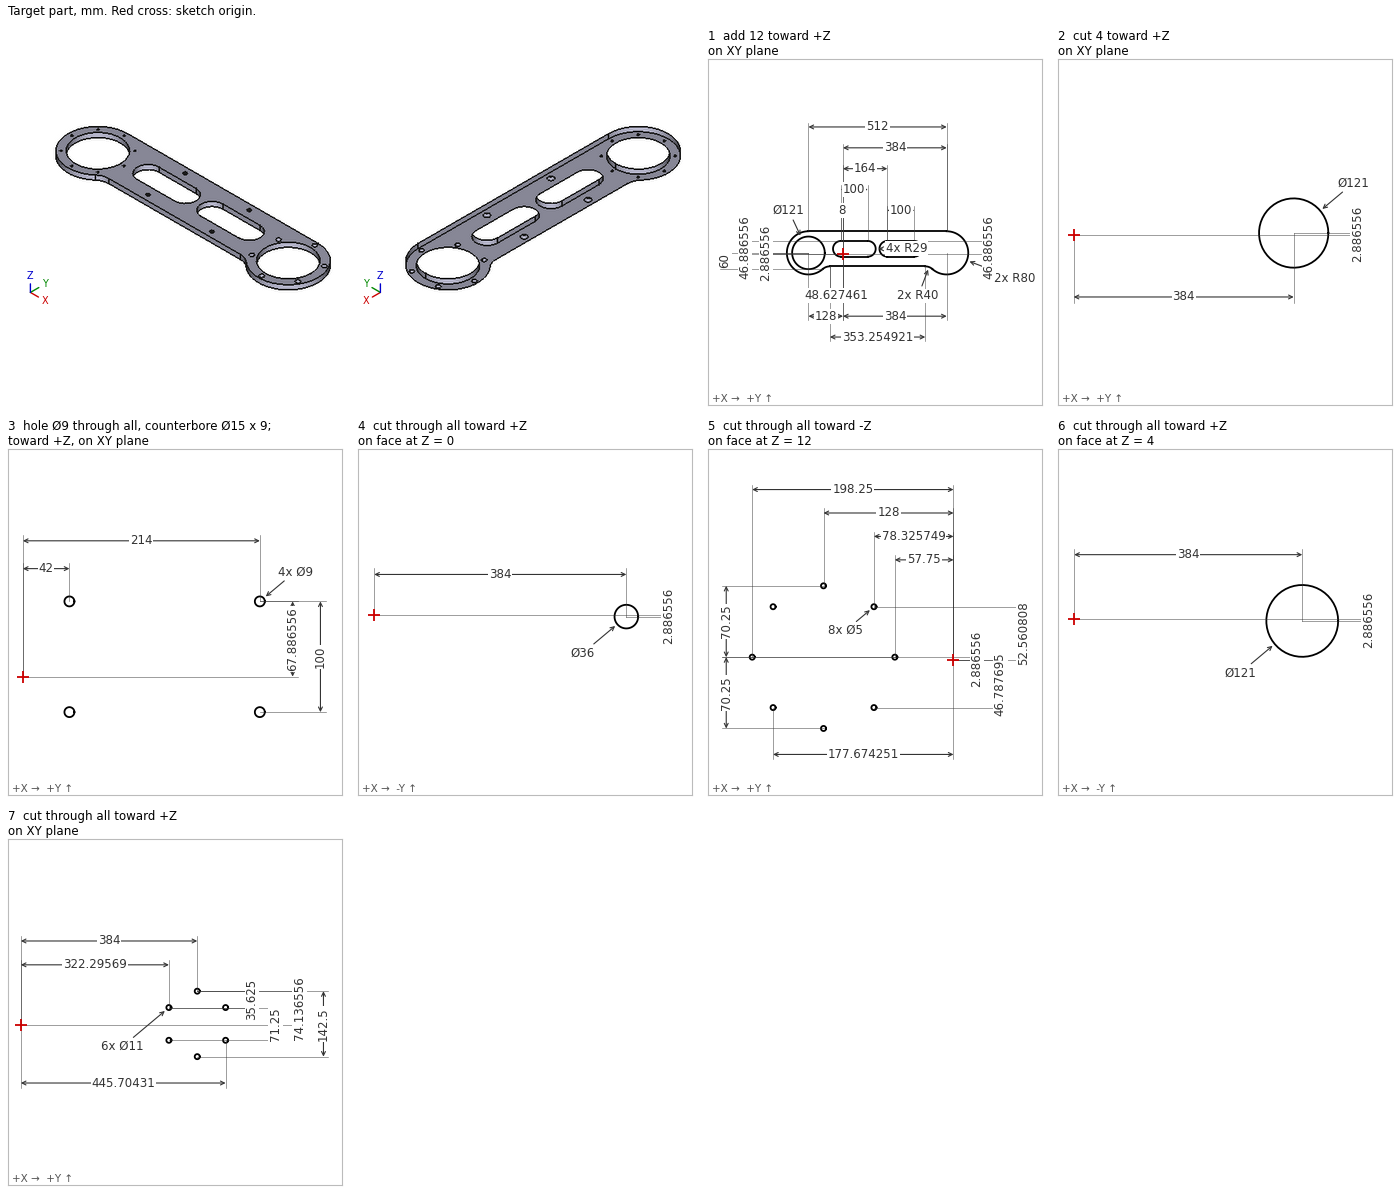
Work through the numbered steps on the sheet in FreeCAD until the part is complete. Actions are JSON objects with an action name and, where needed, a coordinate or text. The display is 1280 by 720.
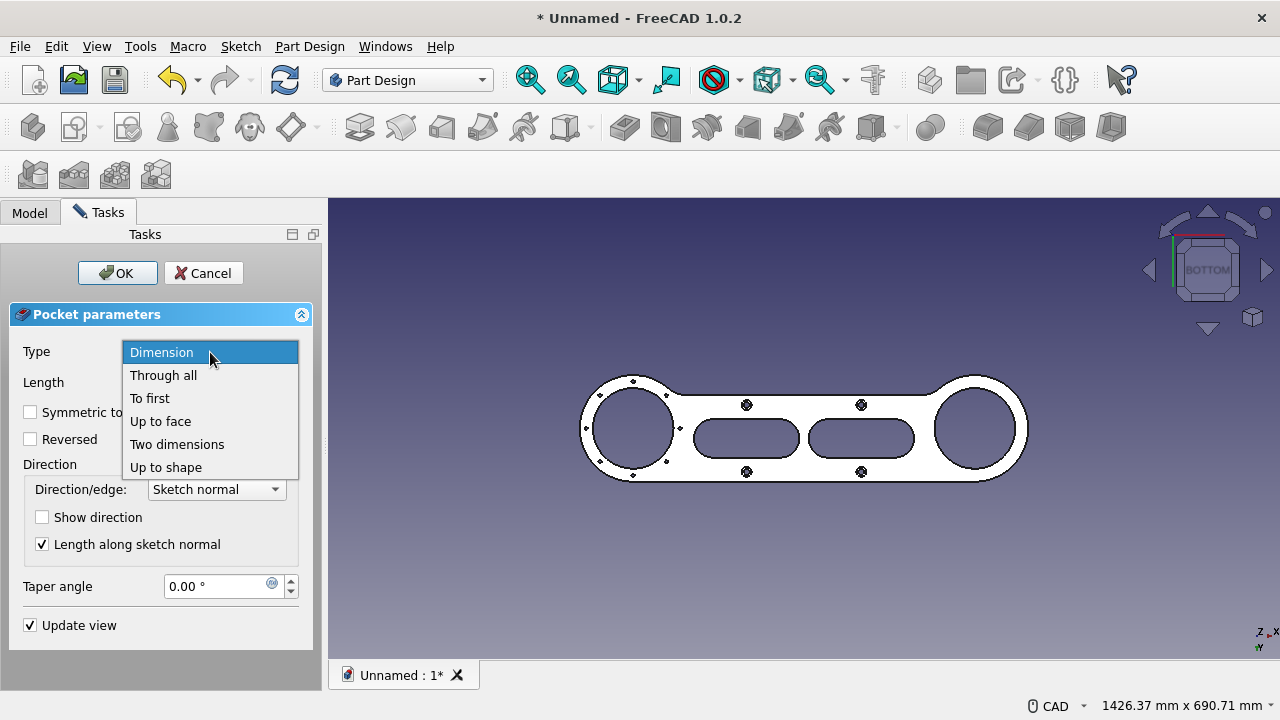
{"action": "left_click", "coordinate": [208, 376]}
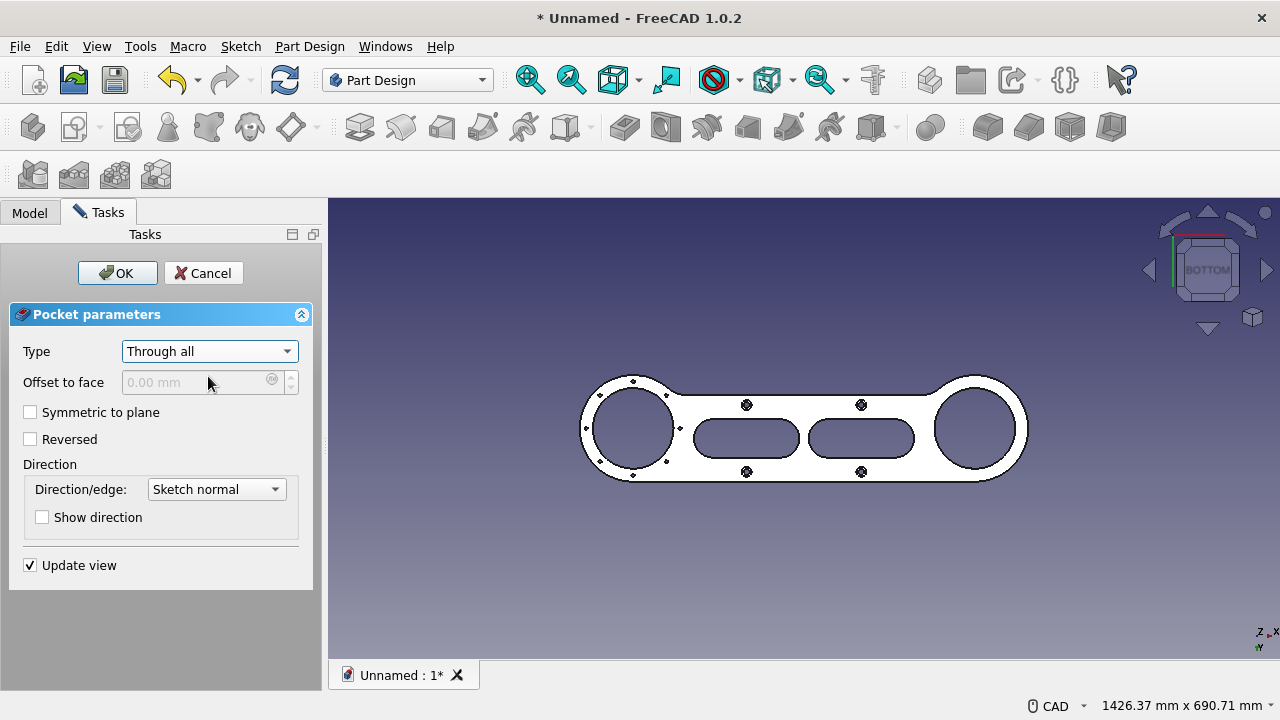
{"action": "left_click", "coordinate": [31, 439]}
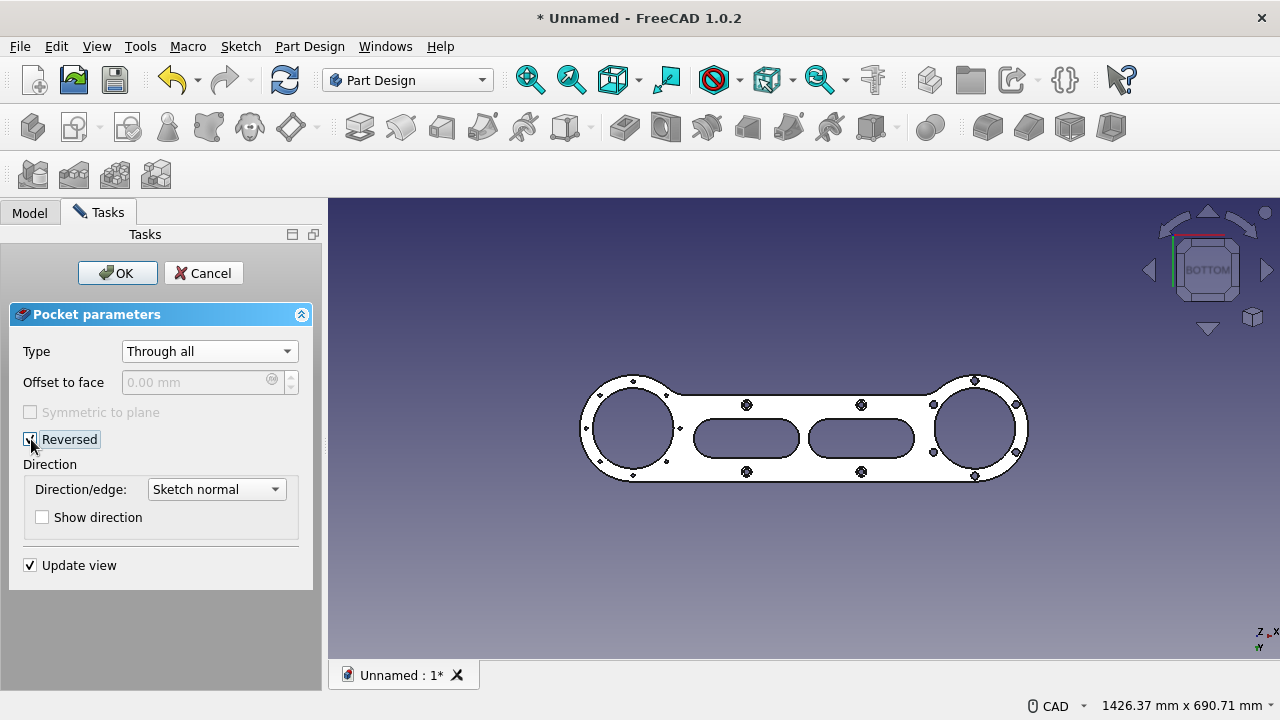
{"action": "left_click", "coordinate": [118, 273]}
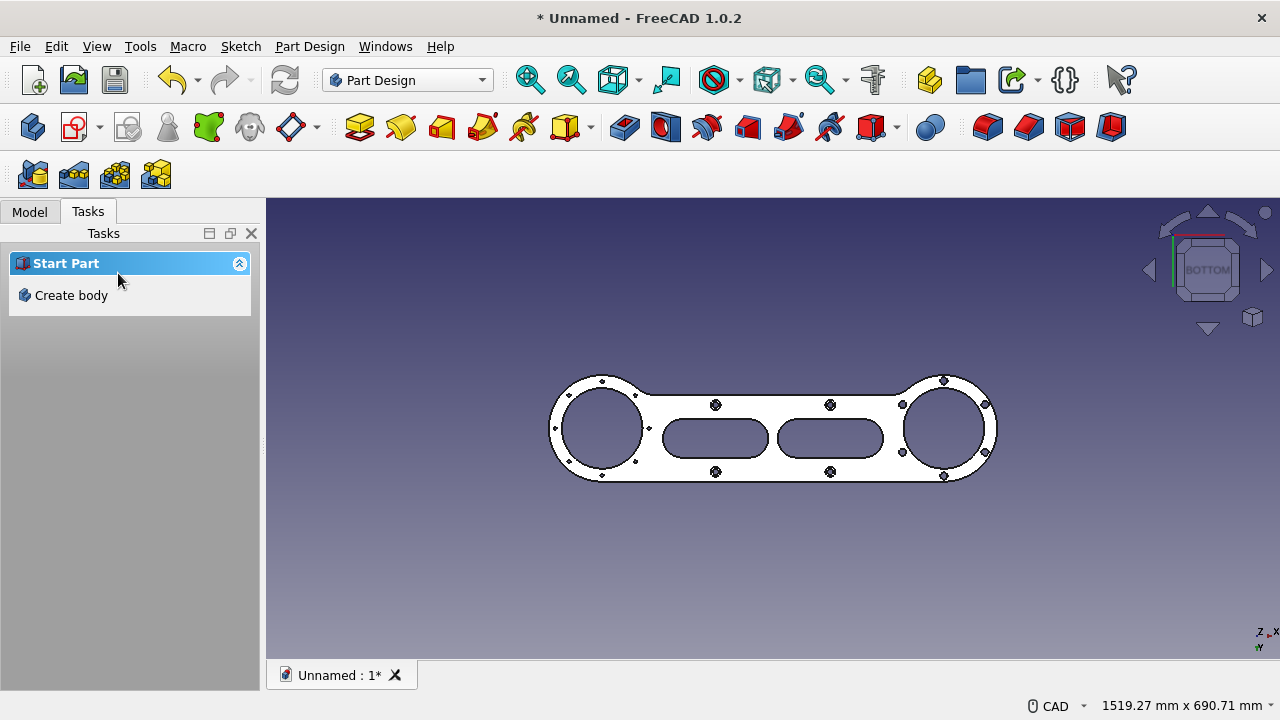
{"action": "key", "text": "0"}